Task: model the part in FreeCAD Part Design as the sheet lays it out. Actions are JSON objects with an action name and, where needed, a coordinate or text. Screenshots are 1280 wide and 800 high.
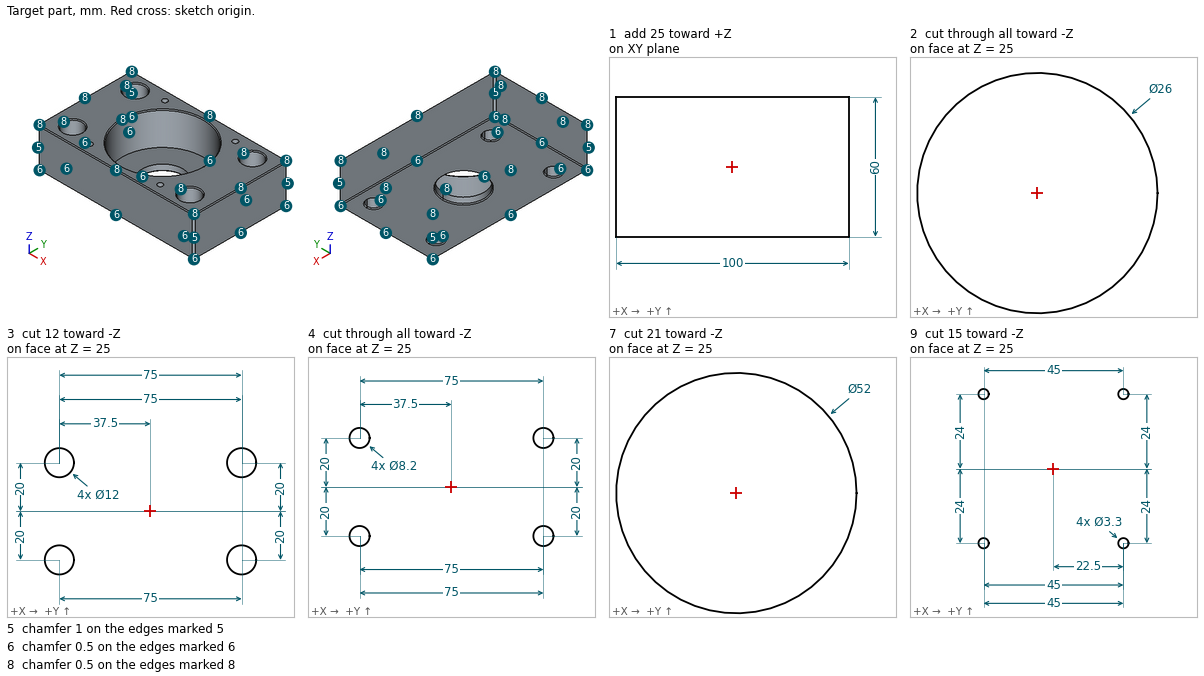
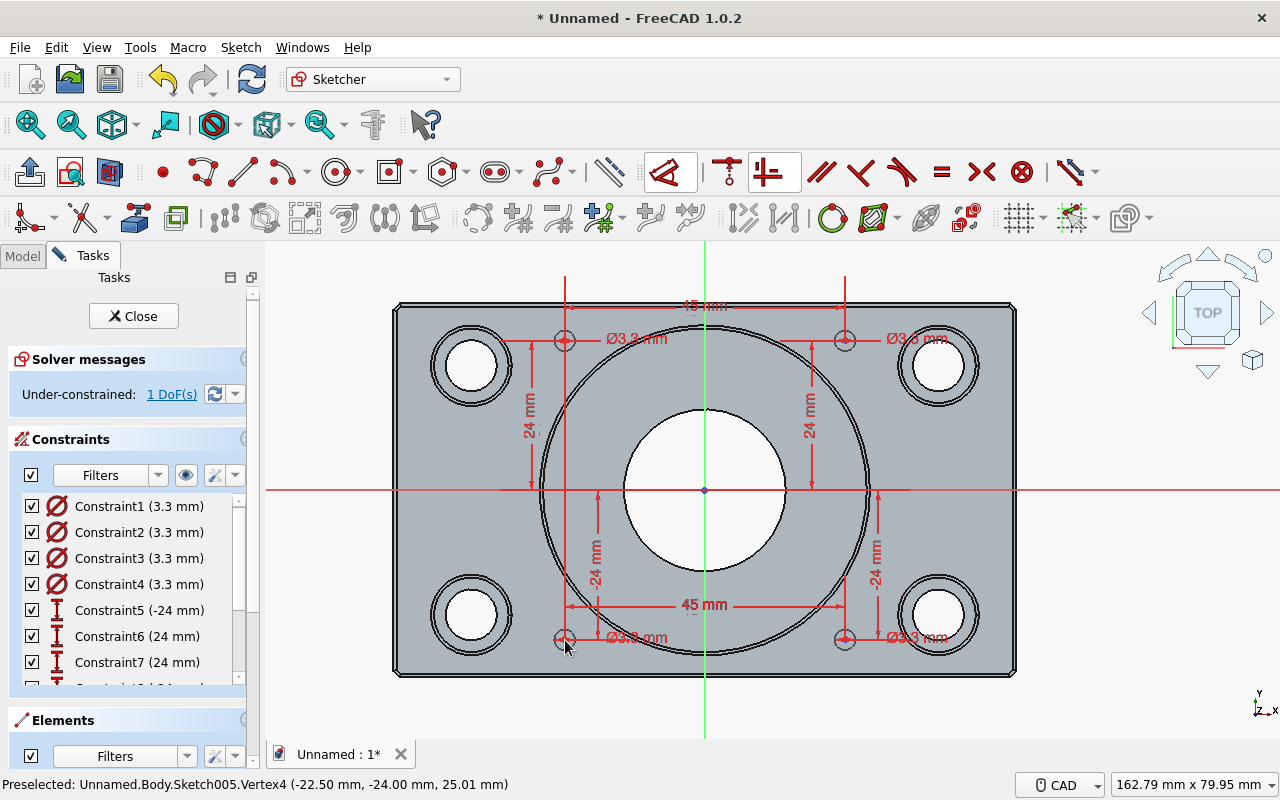
{"action": "left_click", "coordinate": [845, 640]}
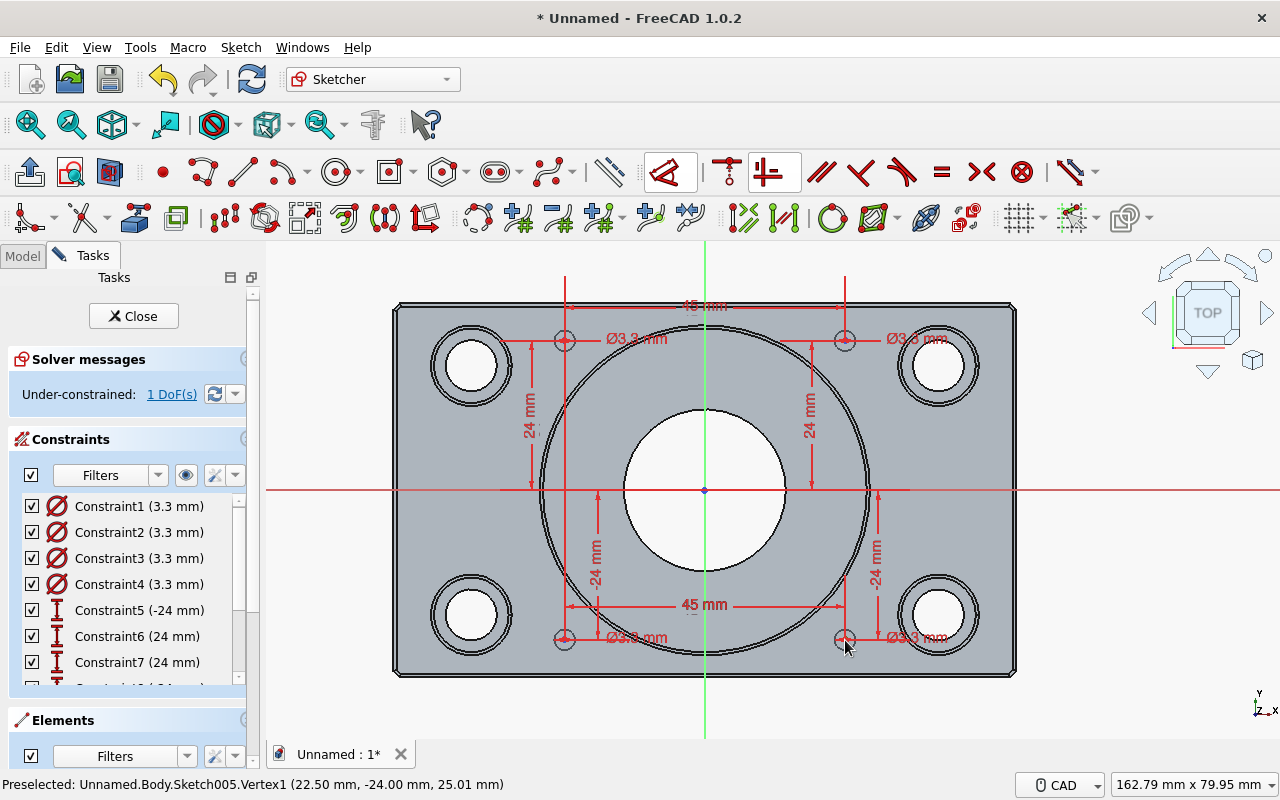
{"action": "key", "text": "l"}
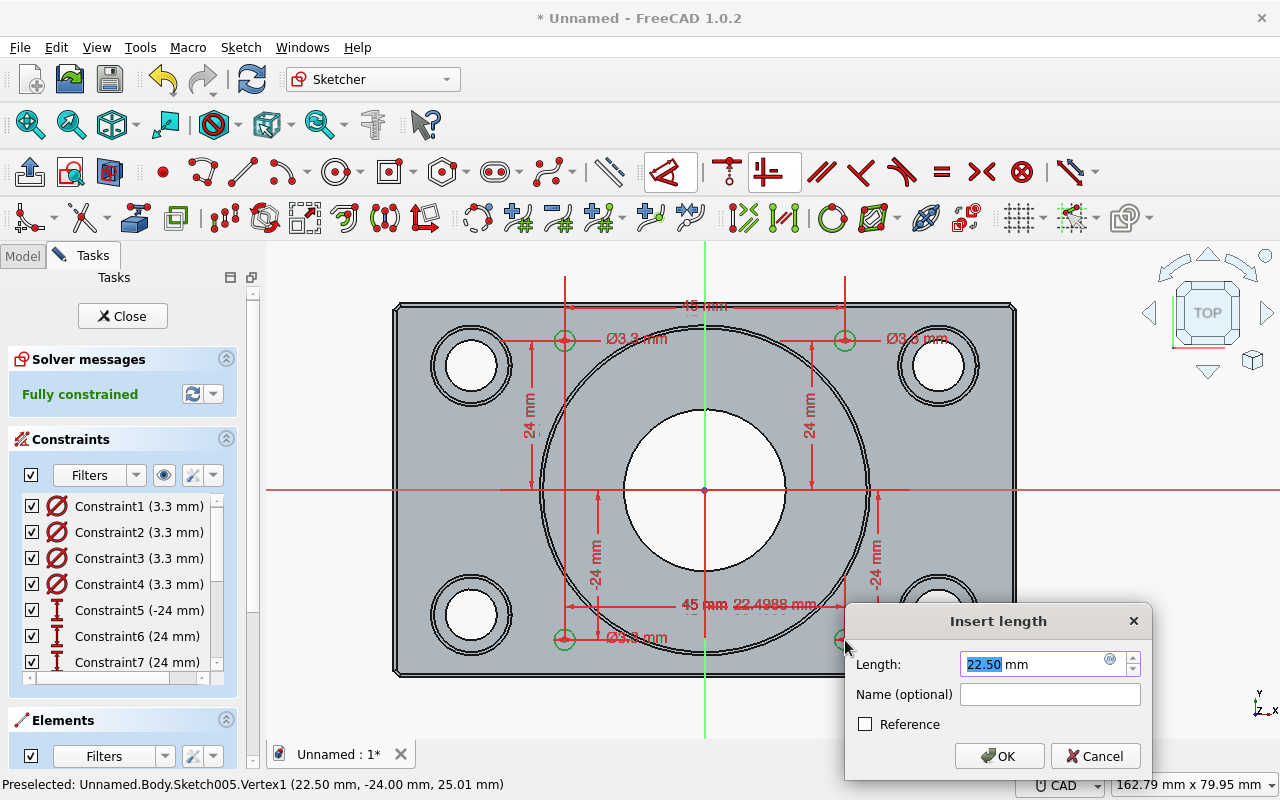
{"action": "type", "text": "22.5"}
{"action": "key", "text": "Return"}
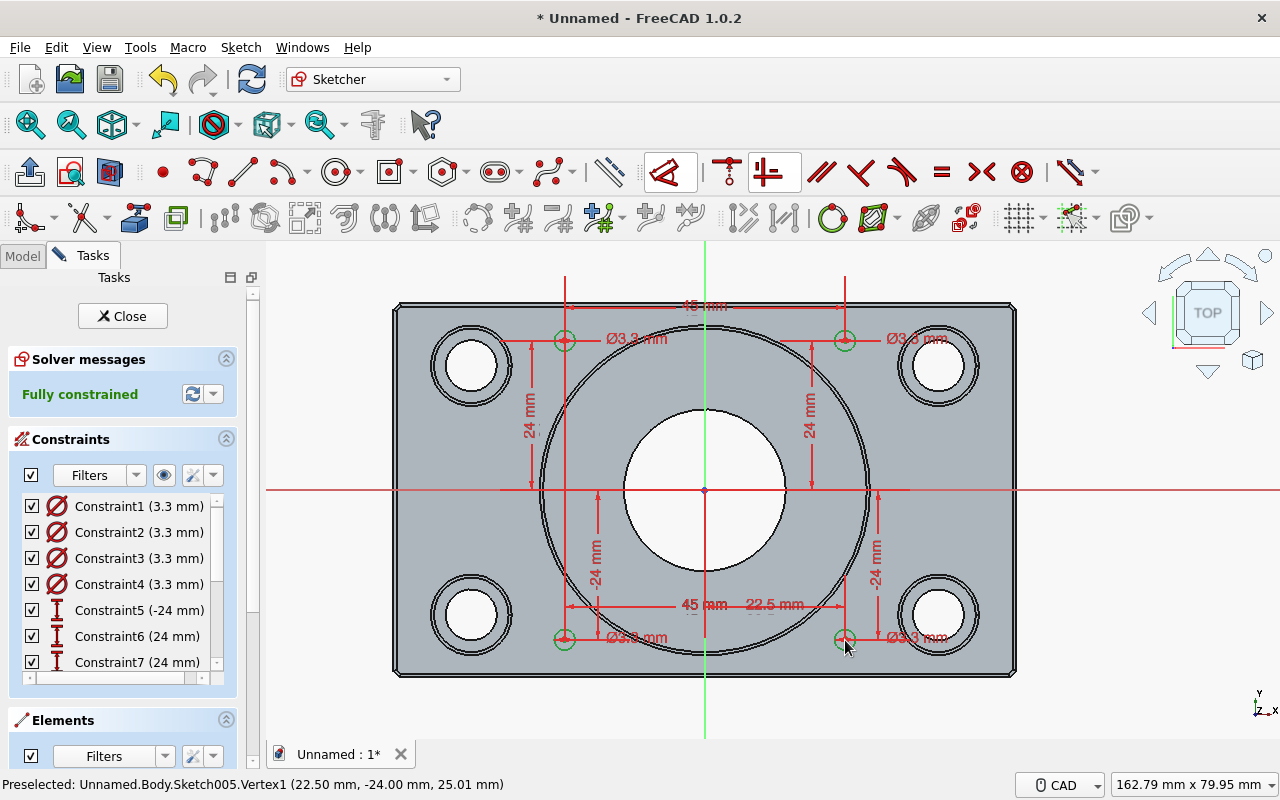
{"action": "left_click", "coordinate": [123, 316]}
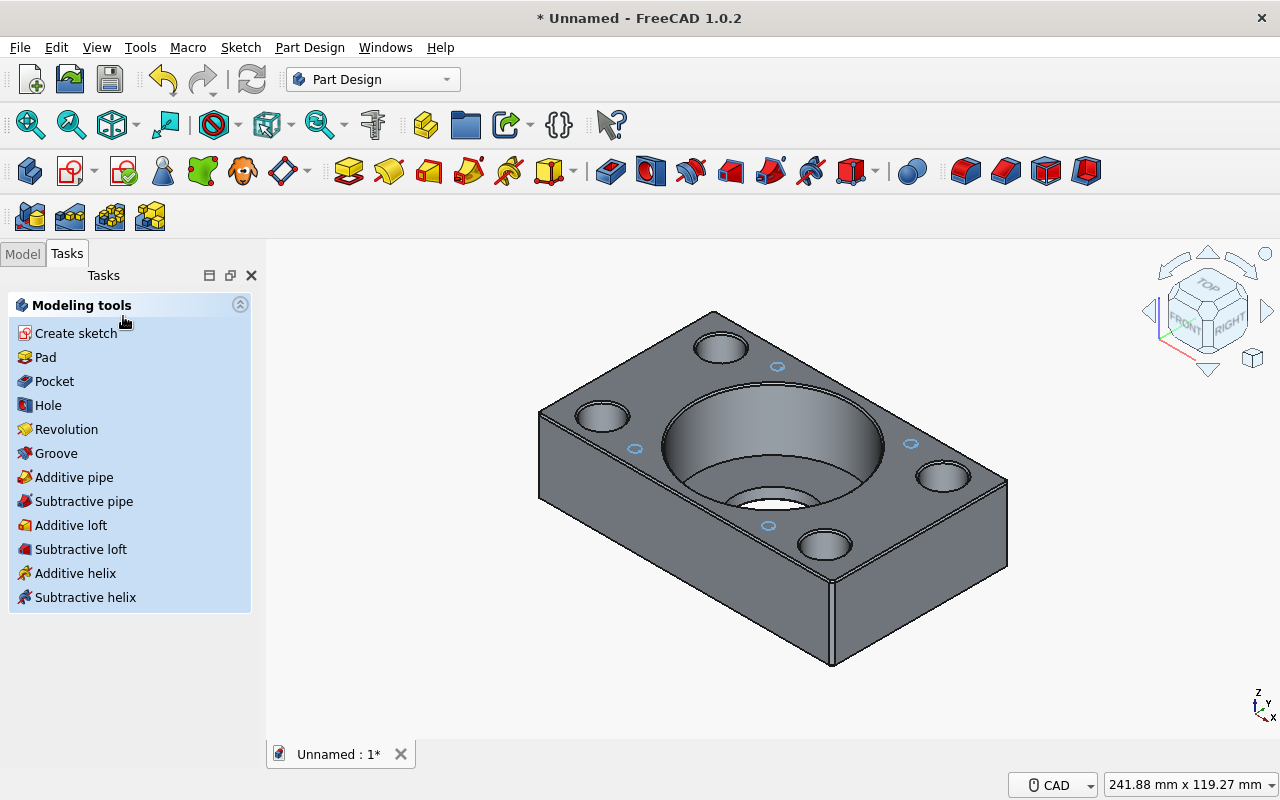
{"action": "left_click", "coordinate": [612, 172]}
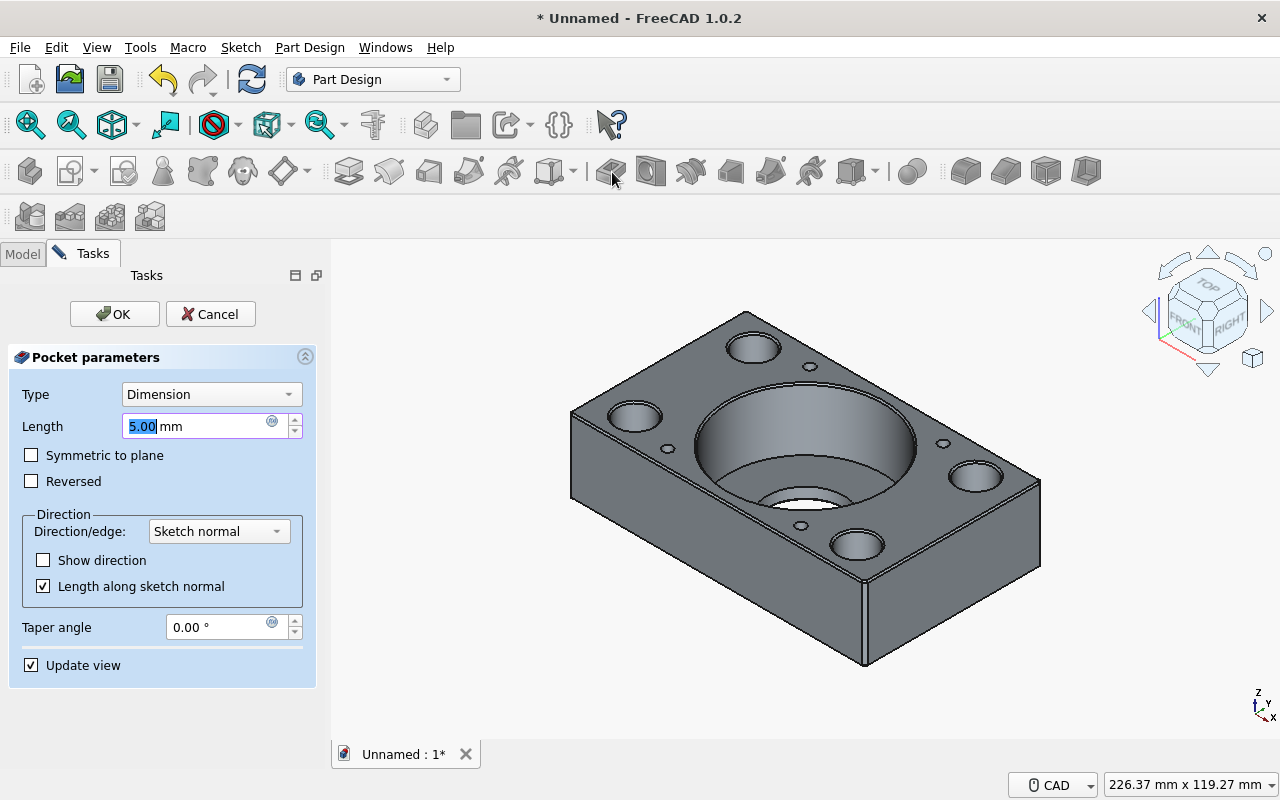
{"action": "type", "text": "15"}
{"action": "key", "text": "Tab"}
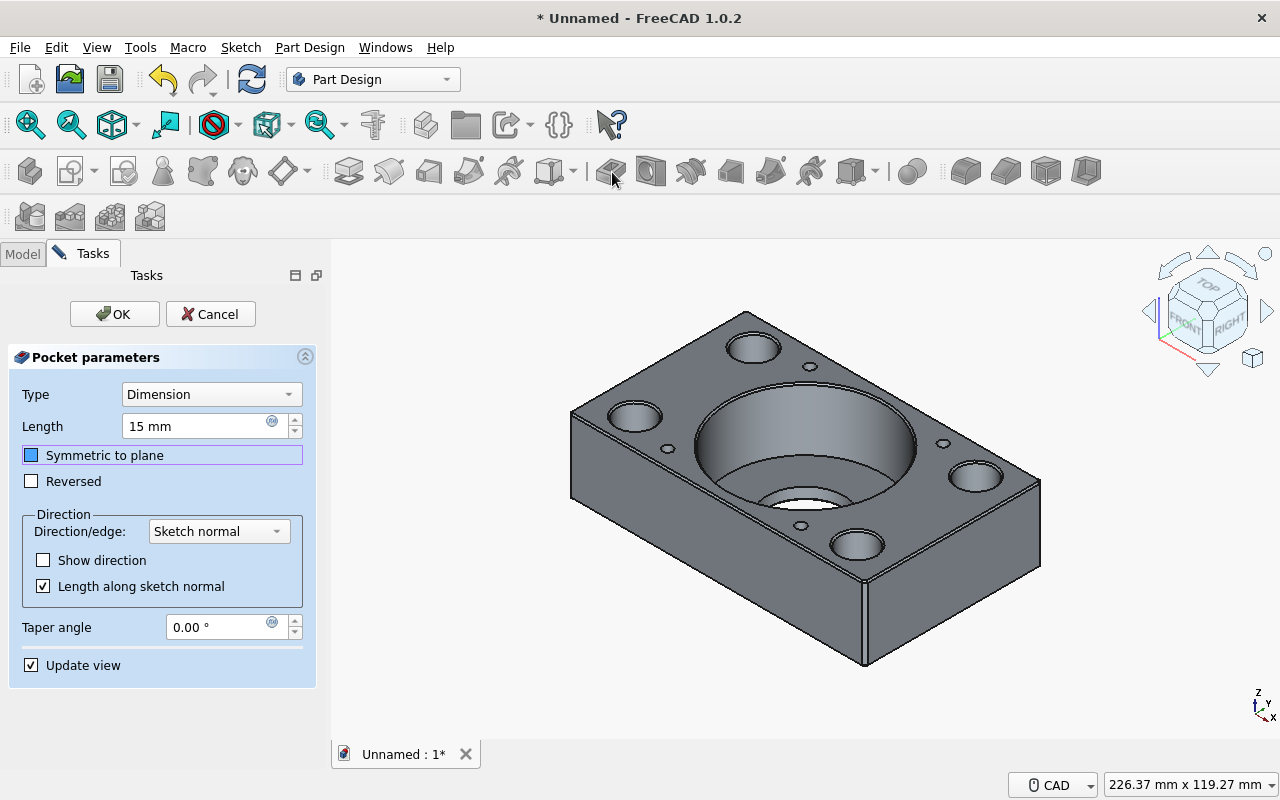
{"action": "left_click", "coordinate": [115, 314]}